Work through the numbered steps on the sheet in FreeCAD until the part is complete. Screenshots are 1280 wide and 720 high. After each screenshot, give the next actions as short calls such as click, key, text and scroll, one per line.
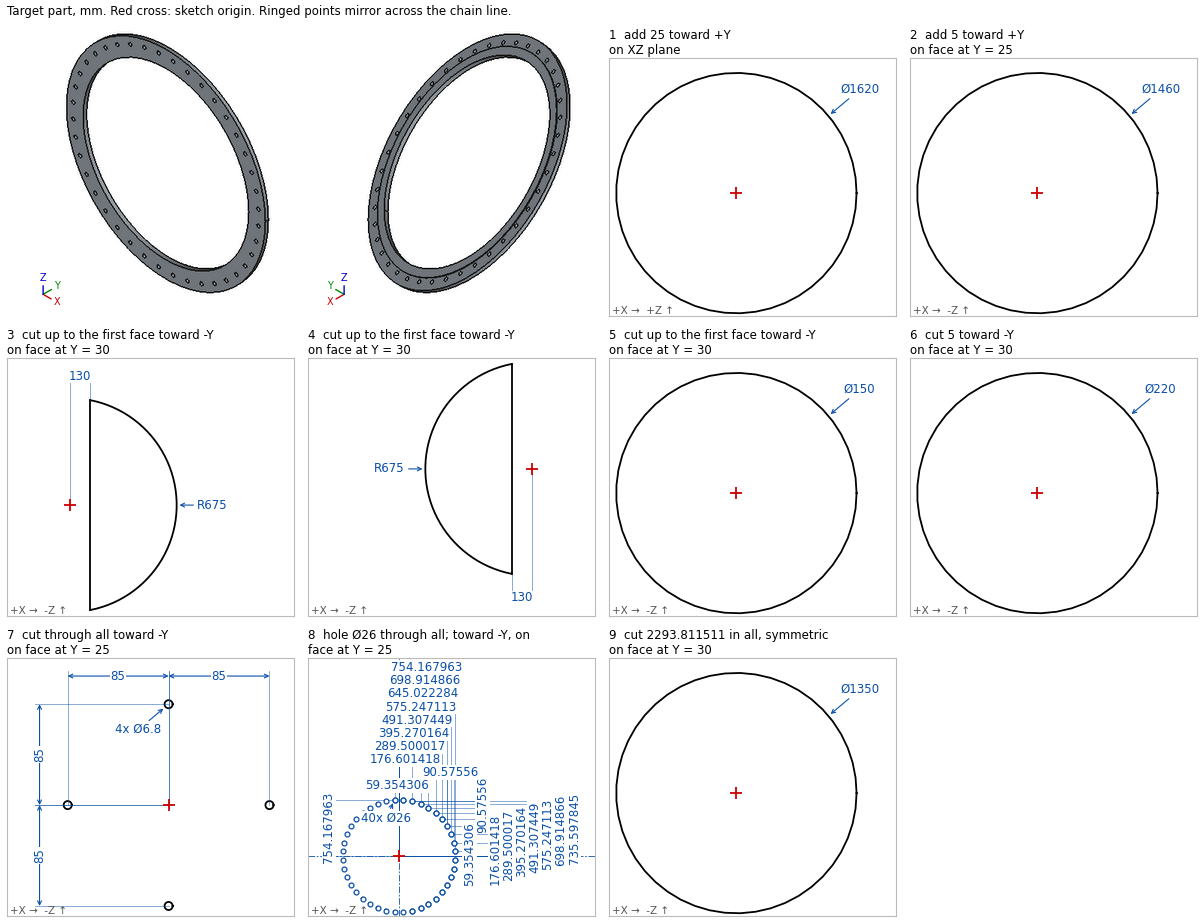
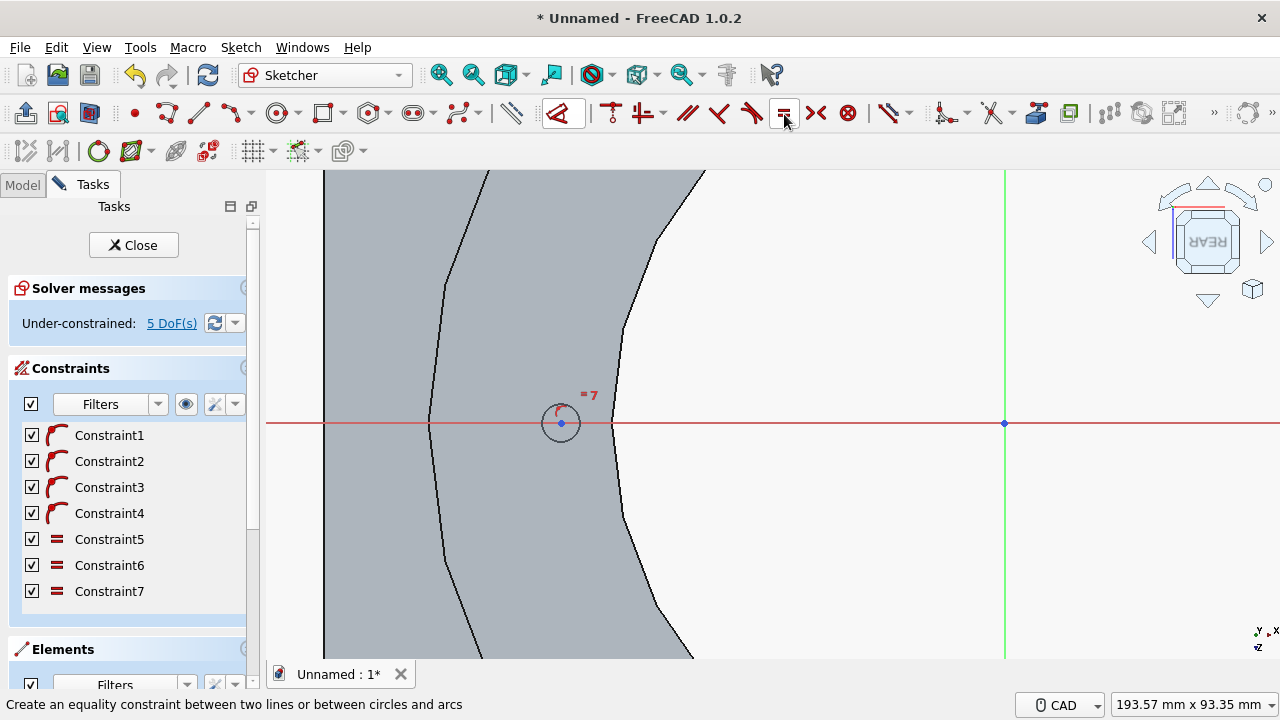
scroll(575, 411, down, 6)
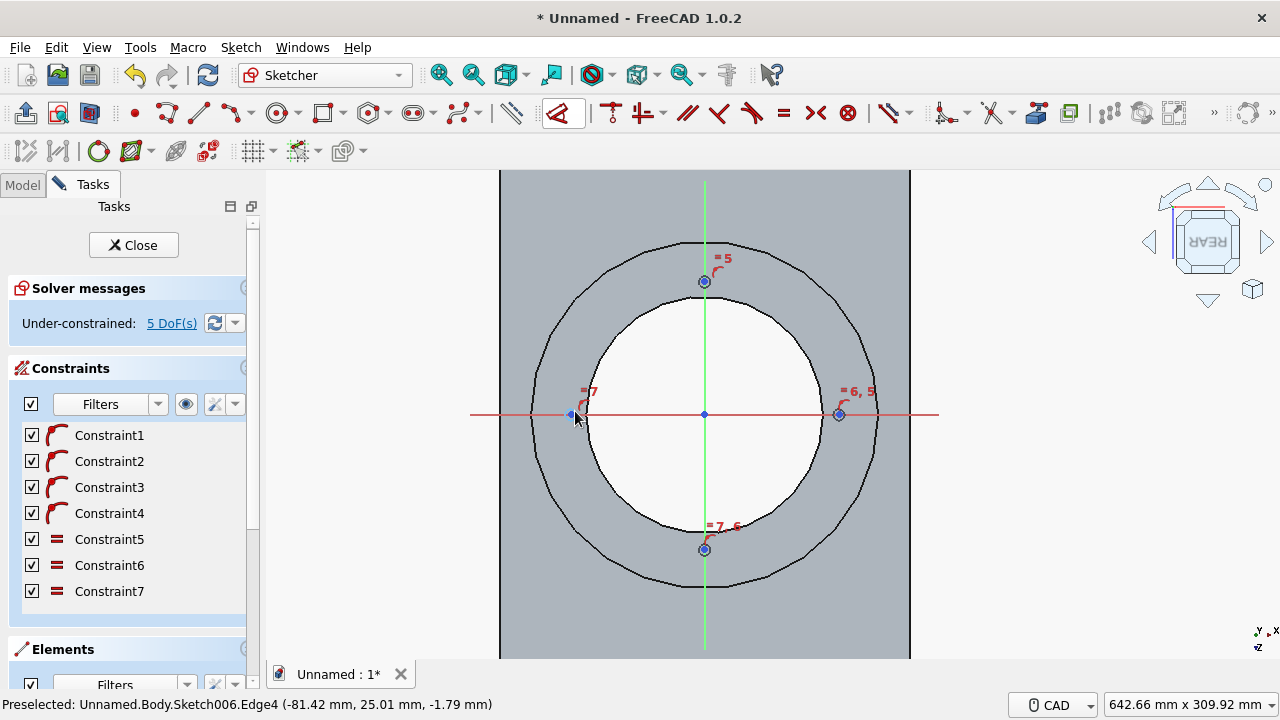
scroll(709, 278, up, 7)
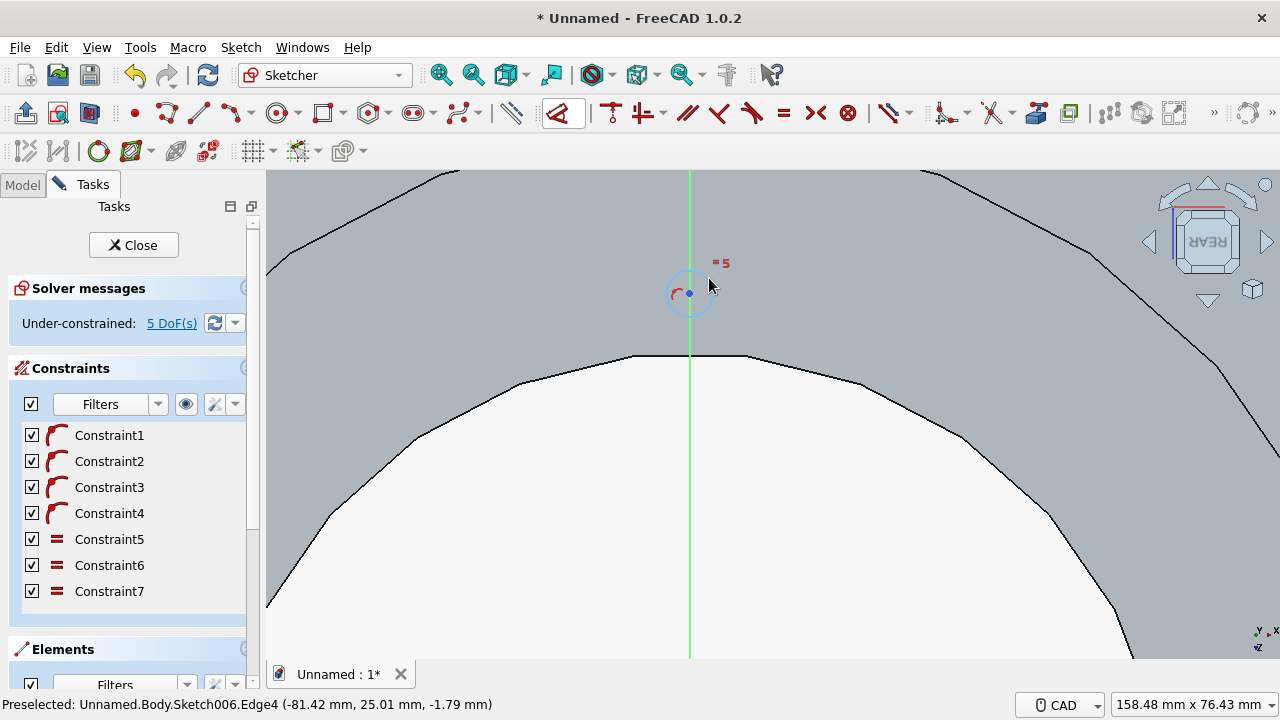
click(706, 277)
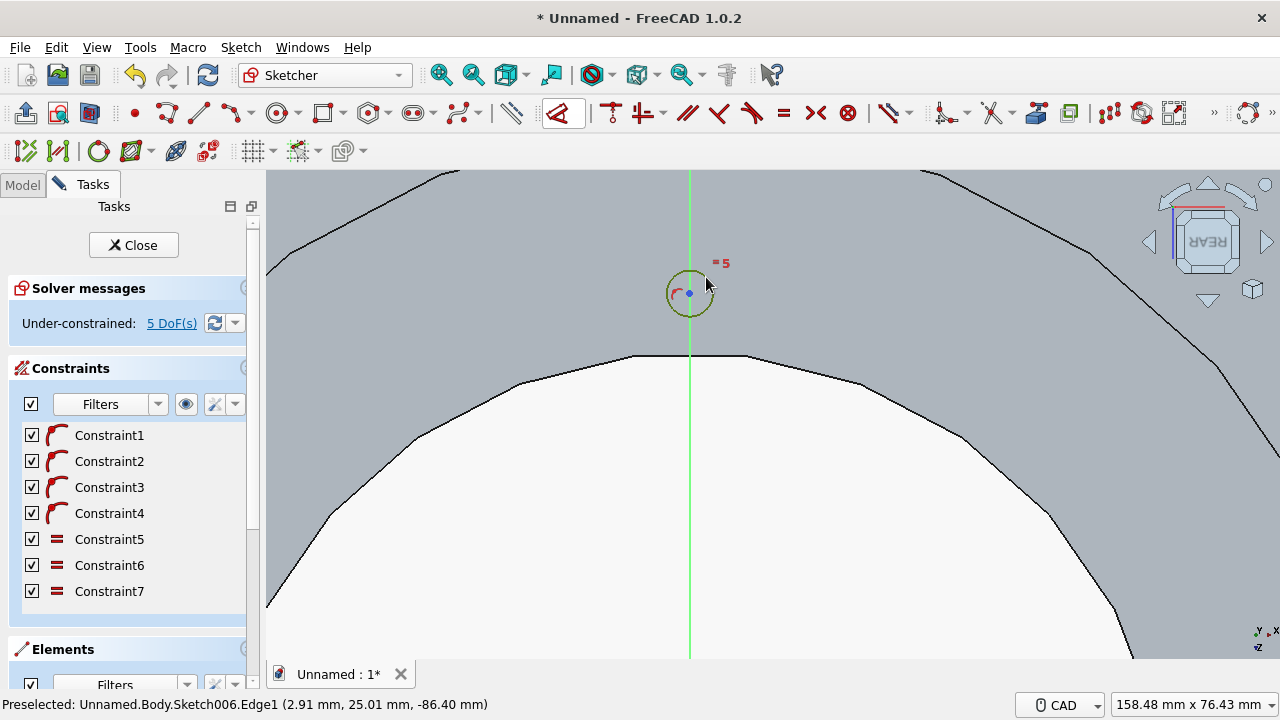
click(580, 114)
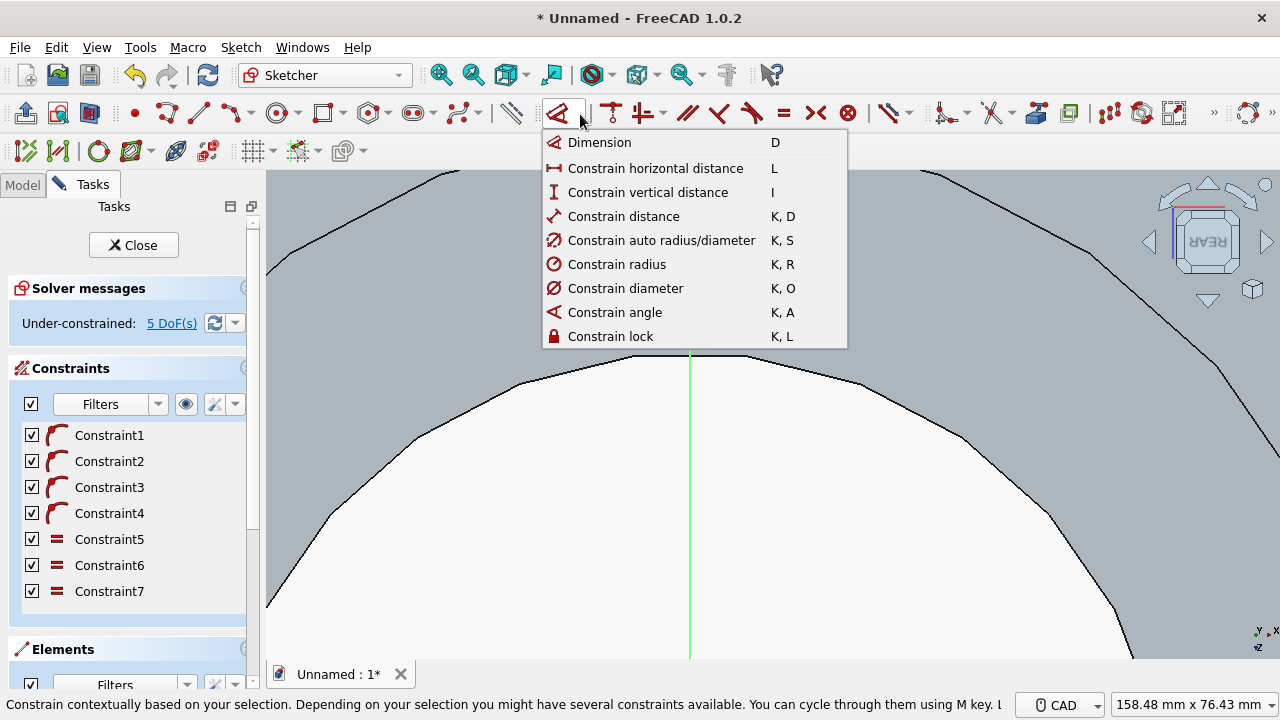
click(695, 288)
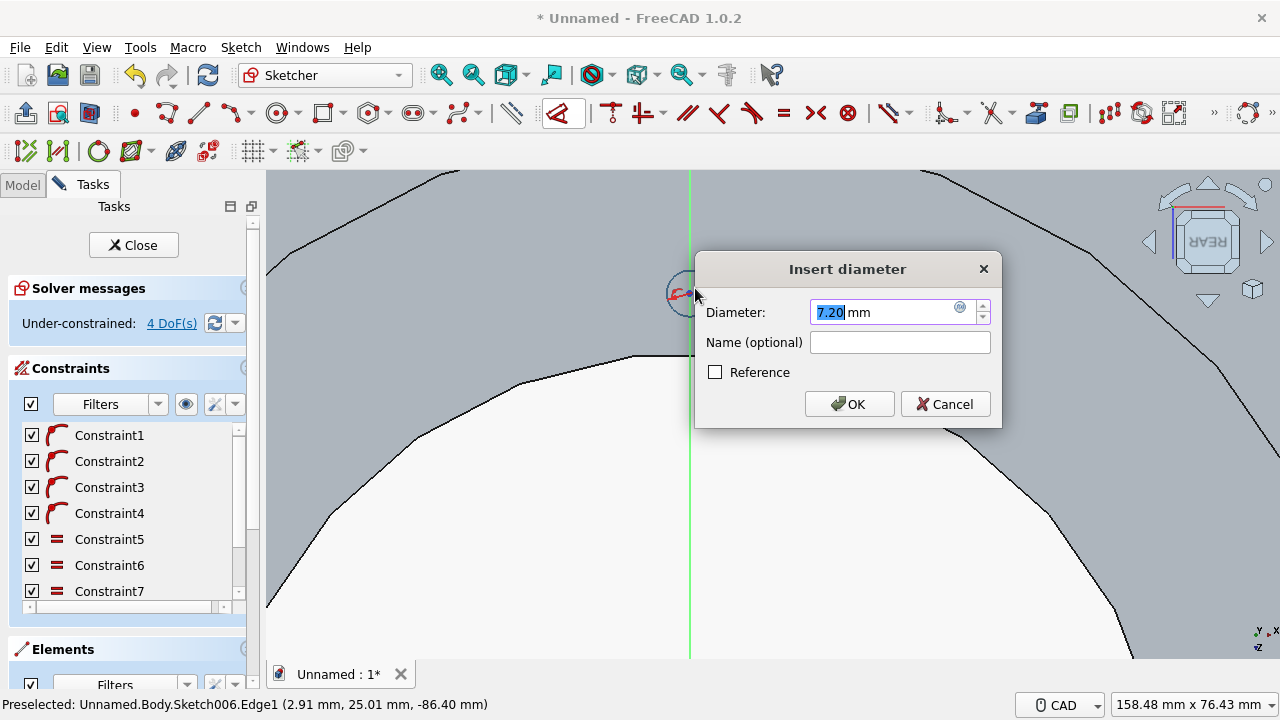
text(6.8)
key(Return)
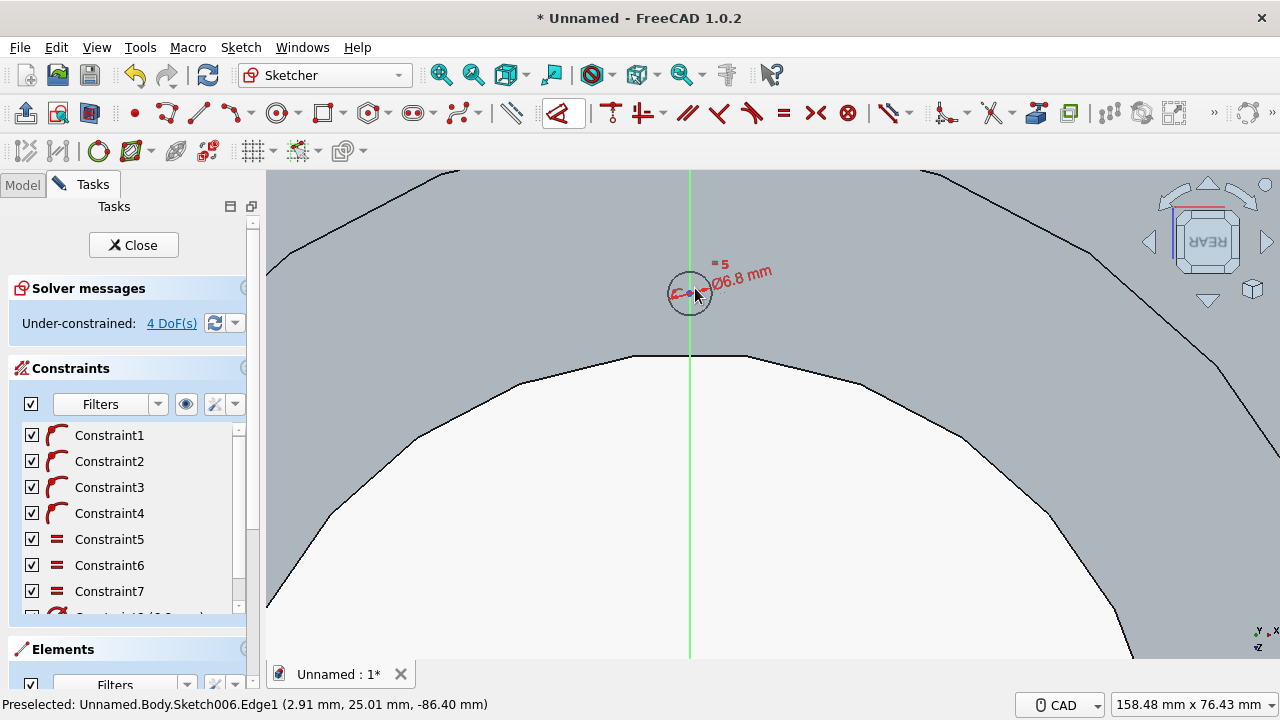
scroll(709, 278, down, 7)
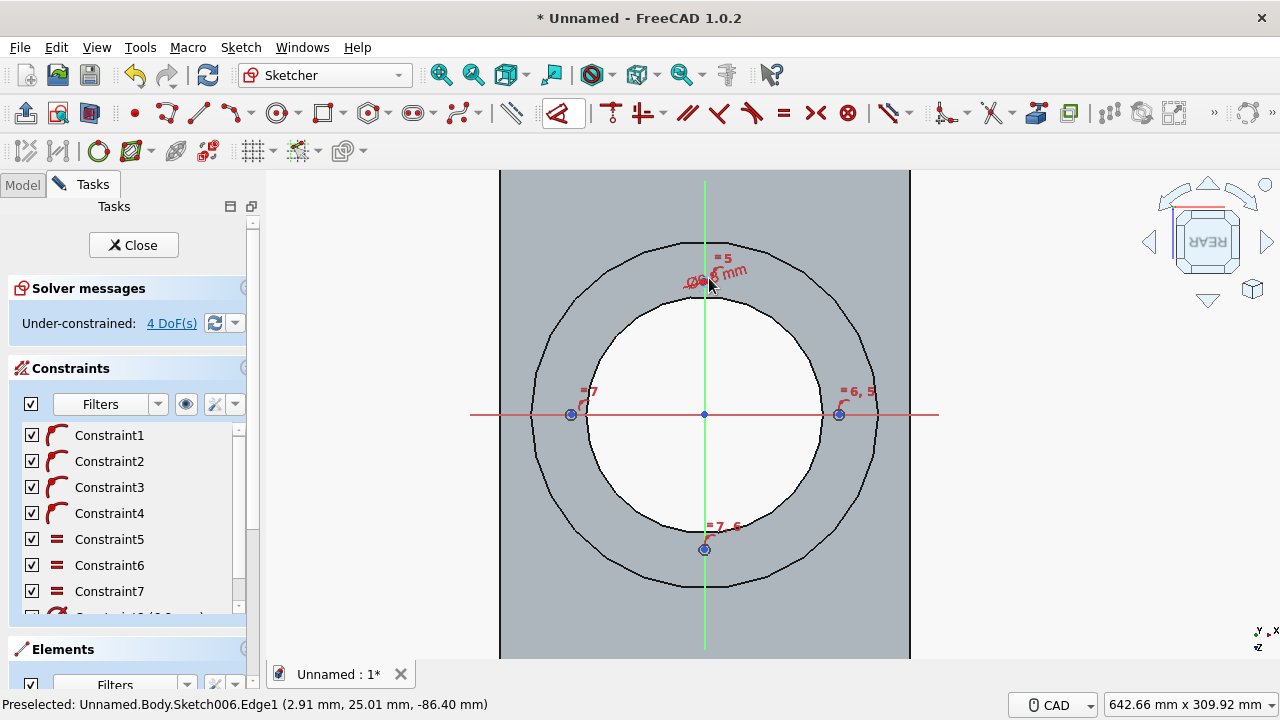
click(705, 282)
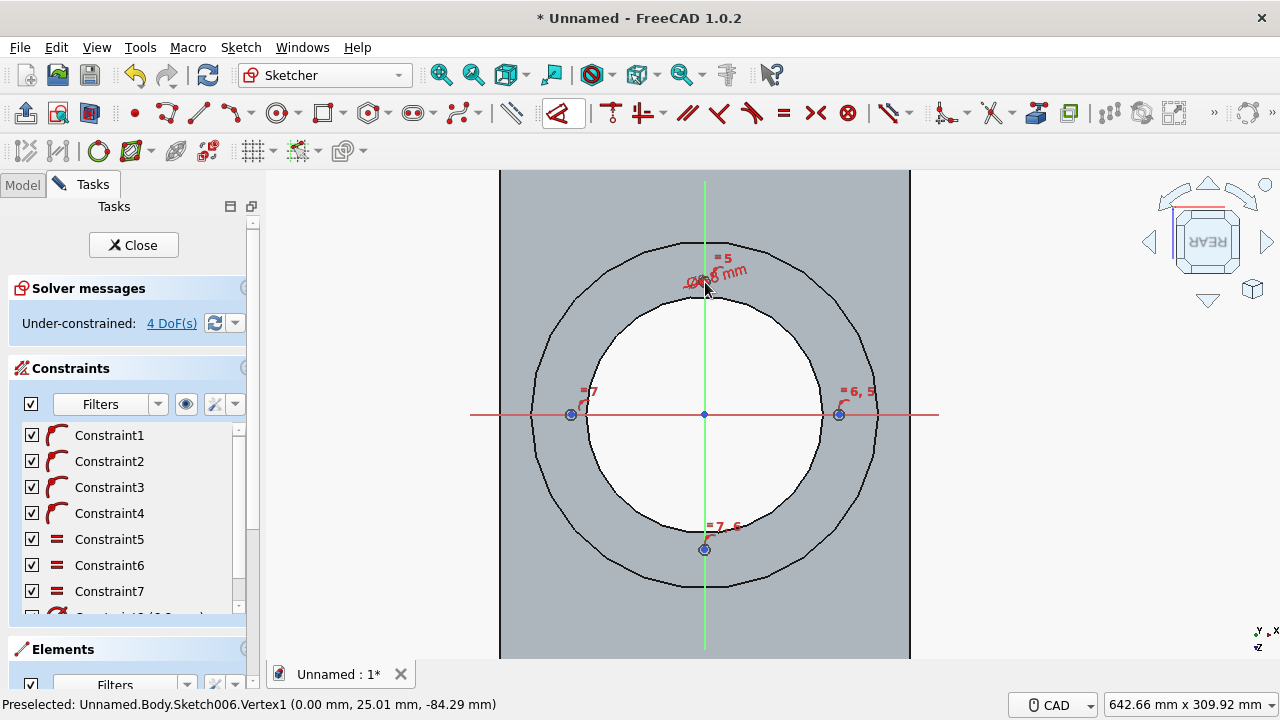
key(i)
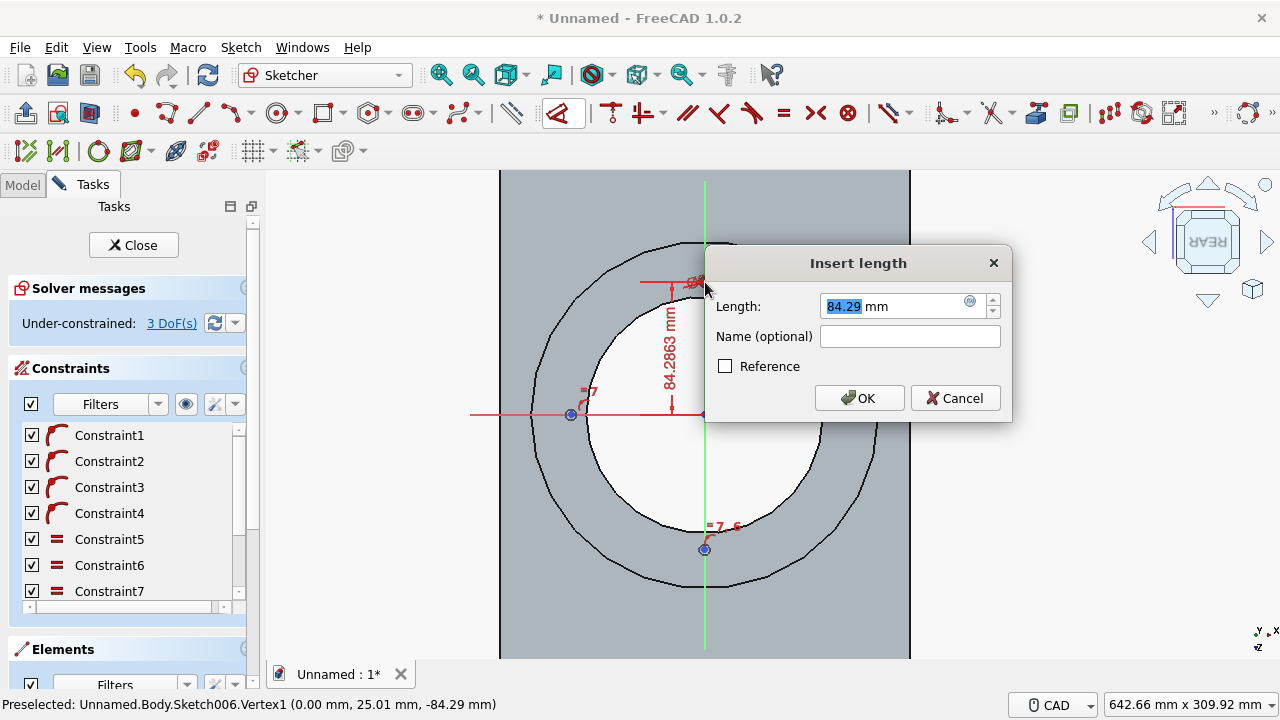
text(85)
key(Return)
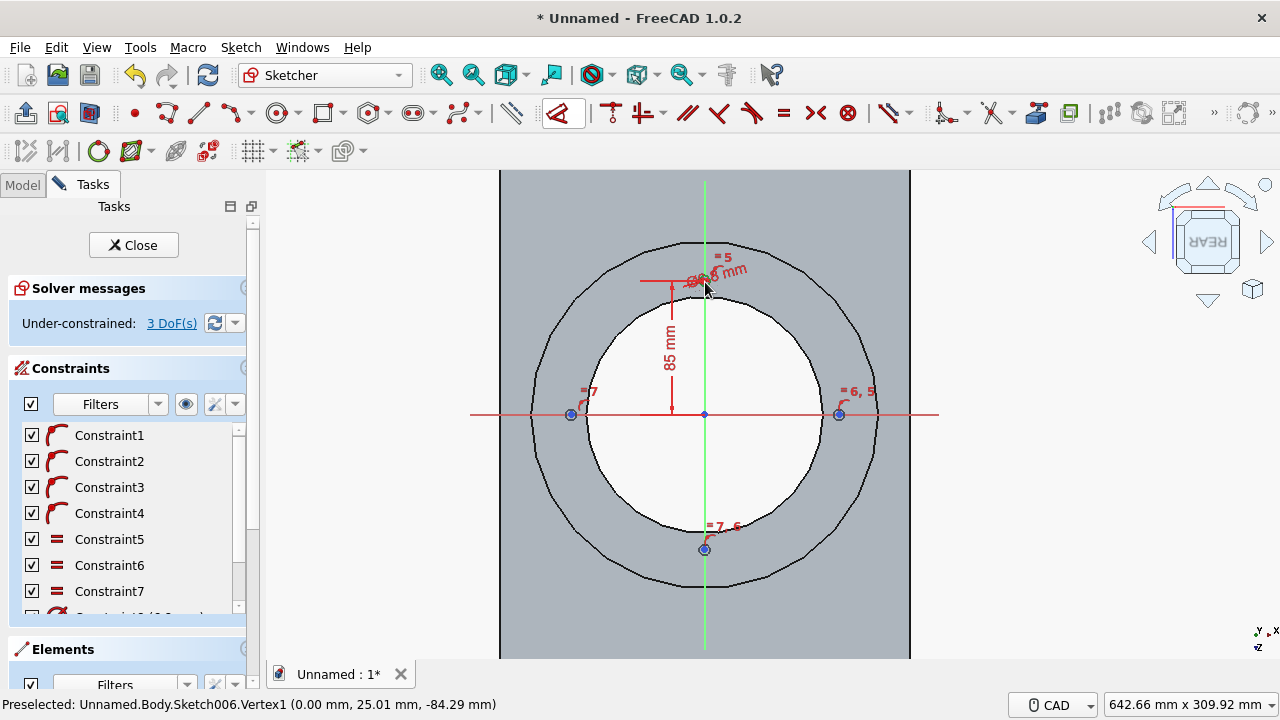
click(839, 415)